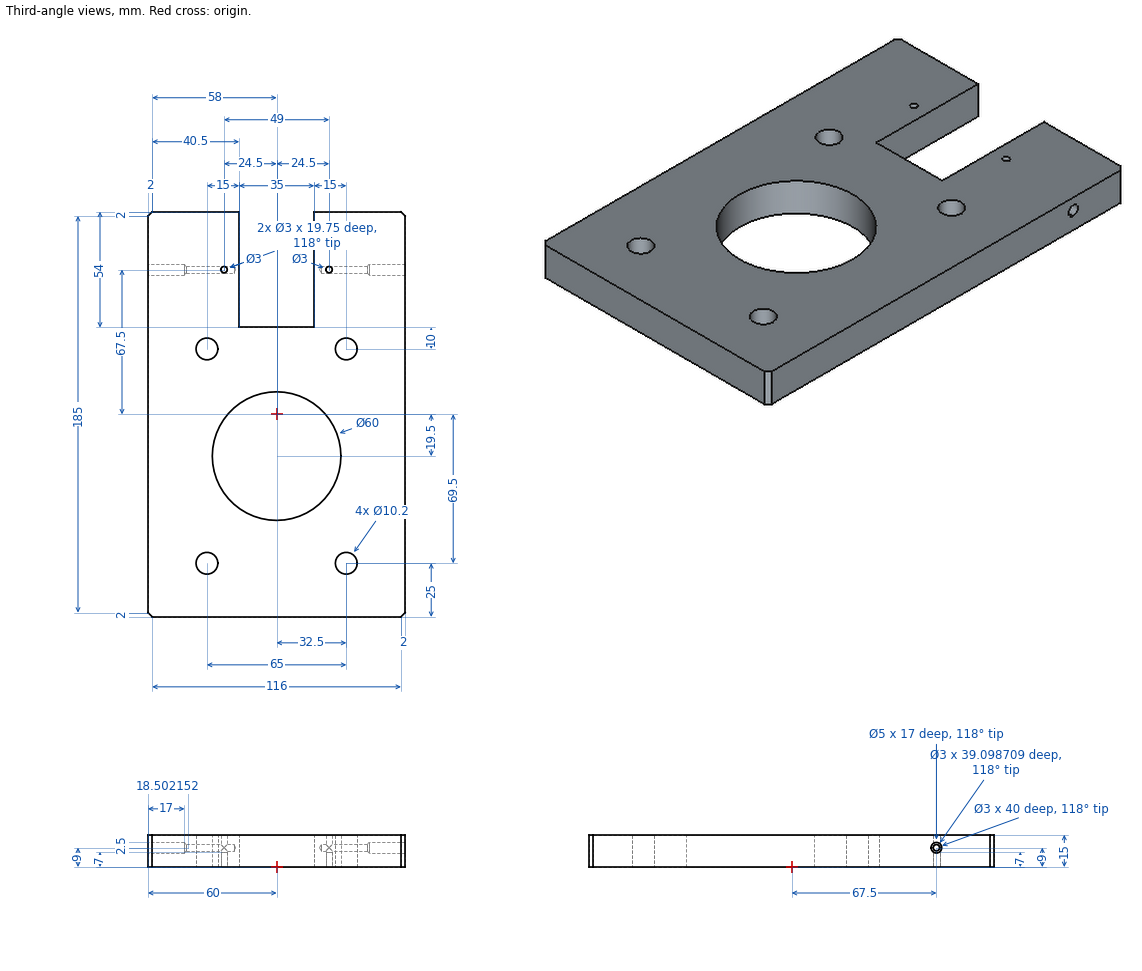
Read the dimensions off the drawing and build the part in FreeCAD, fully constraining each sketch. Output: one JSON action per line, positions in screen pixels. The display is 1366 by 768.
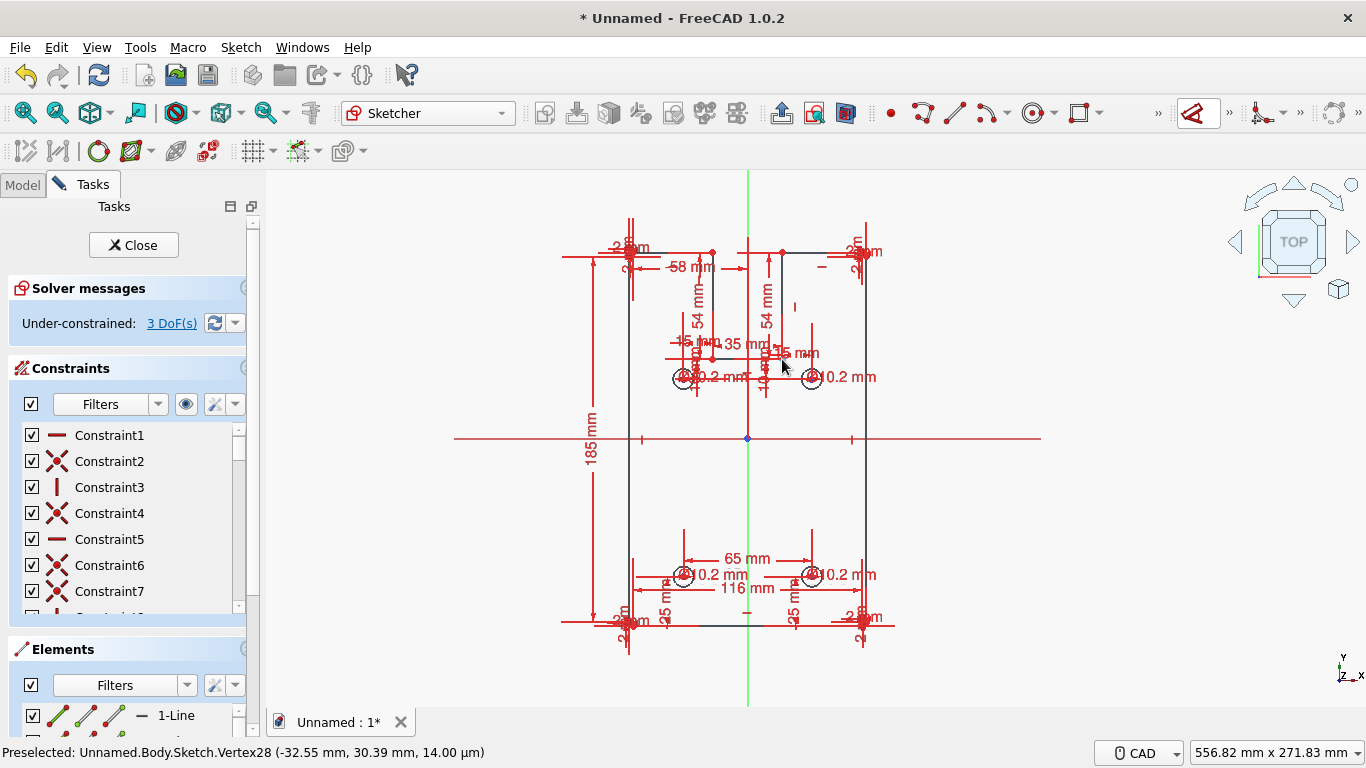
{"action": "left_click", "coordinate": [689, 253]}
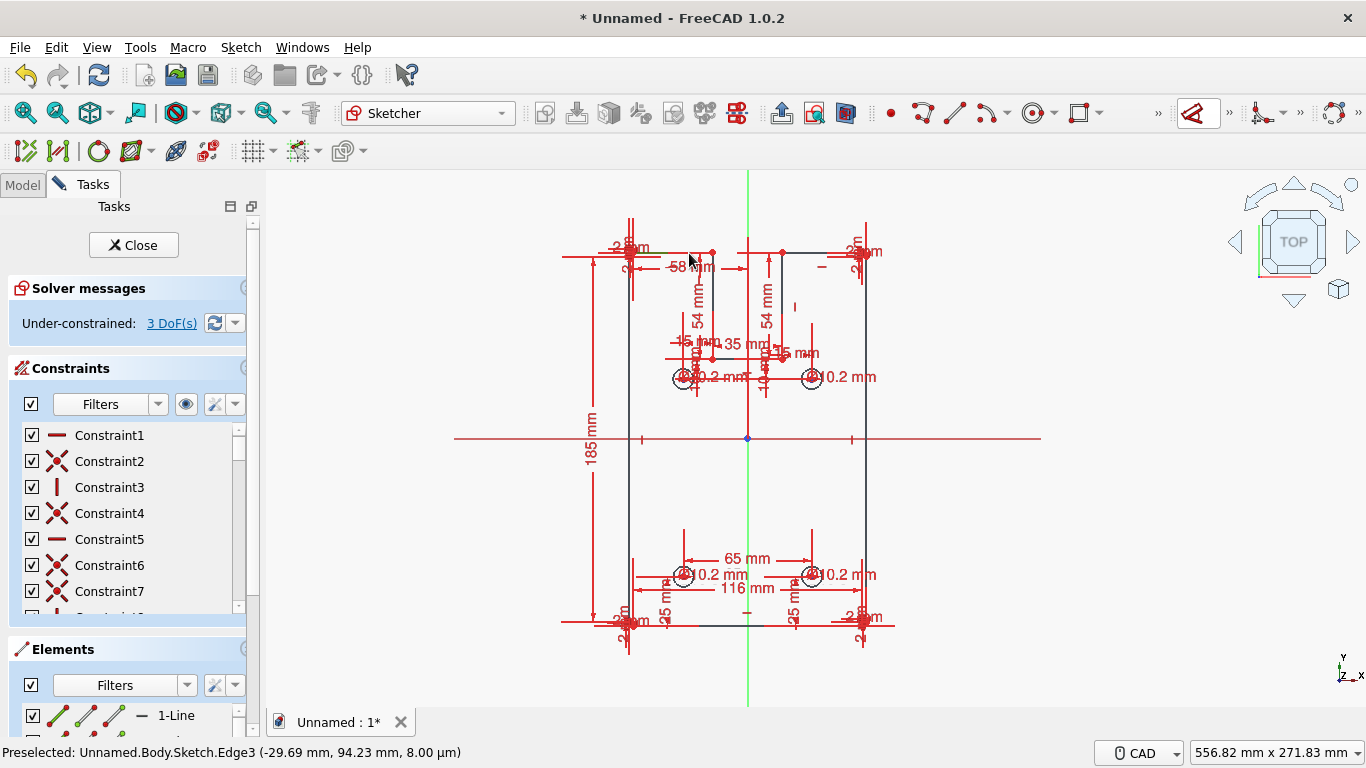
{"action": "key", "text": "l"}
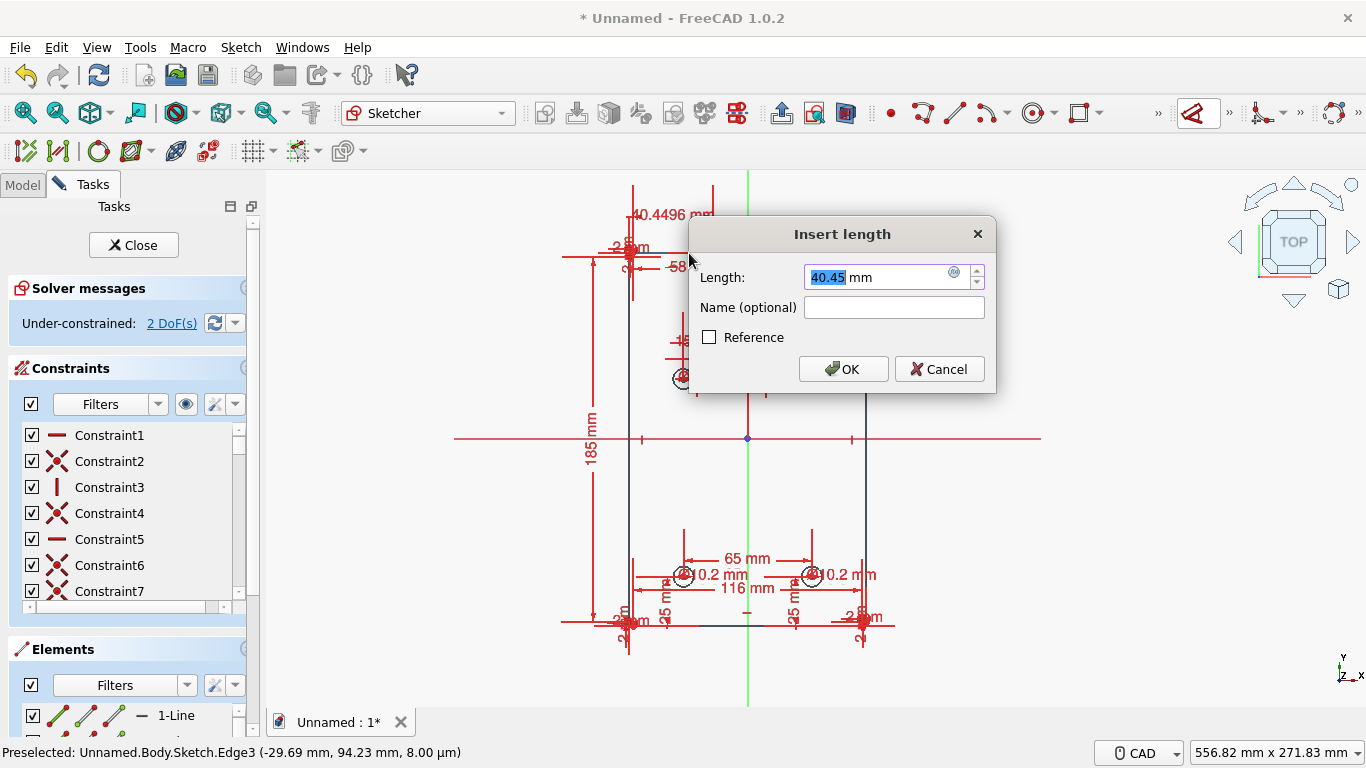
{"action": "type", "text": "40.5"}
{"action": "key", "text": "Return"}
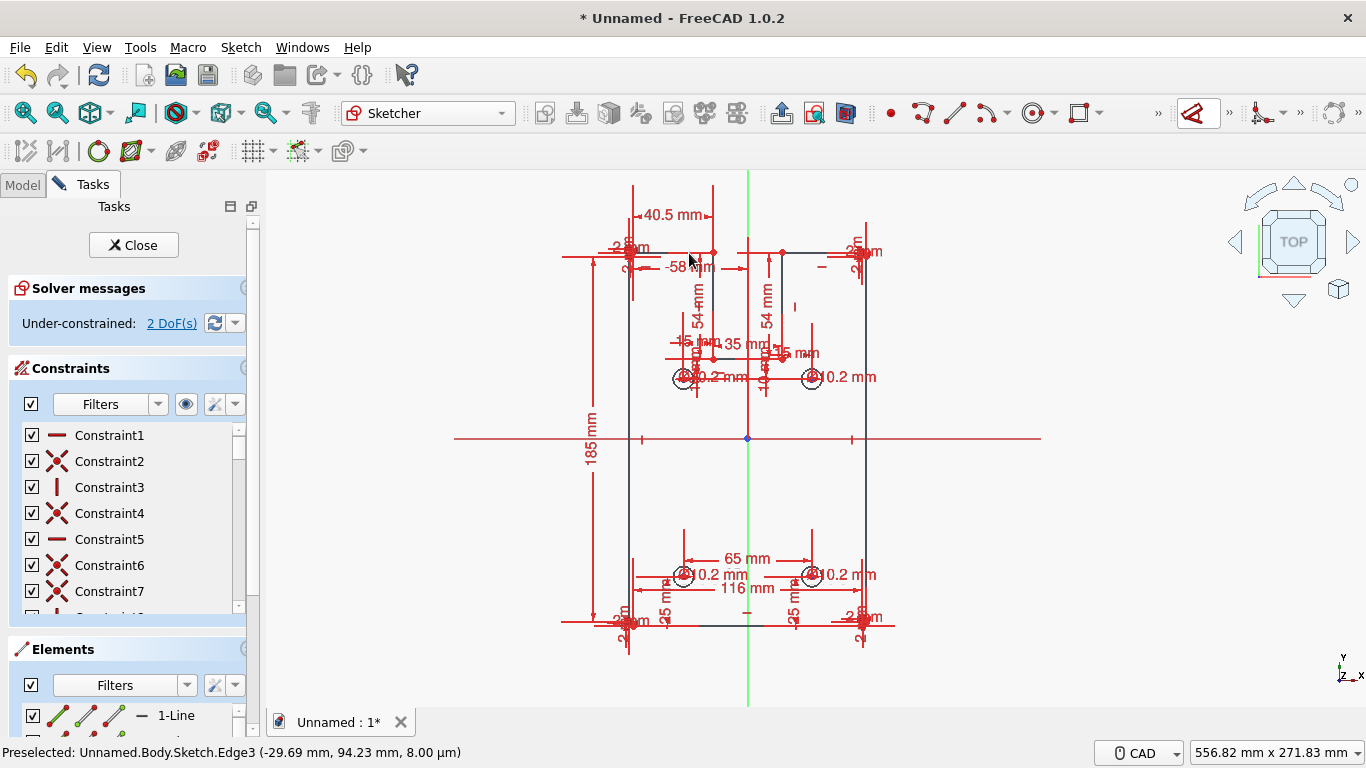
{"action": "left_click", "coordinate": [812, 577]}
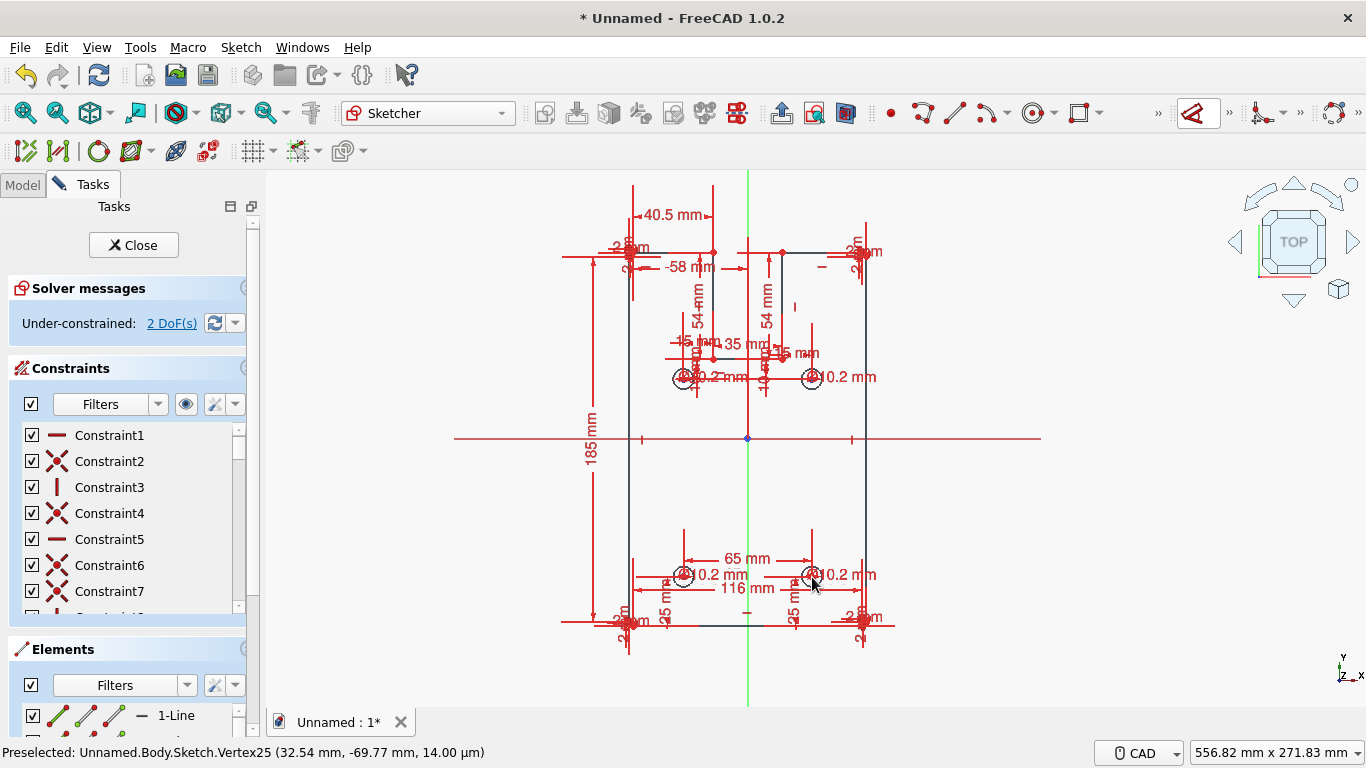
{"action": "key", "text": "l"}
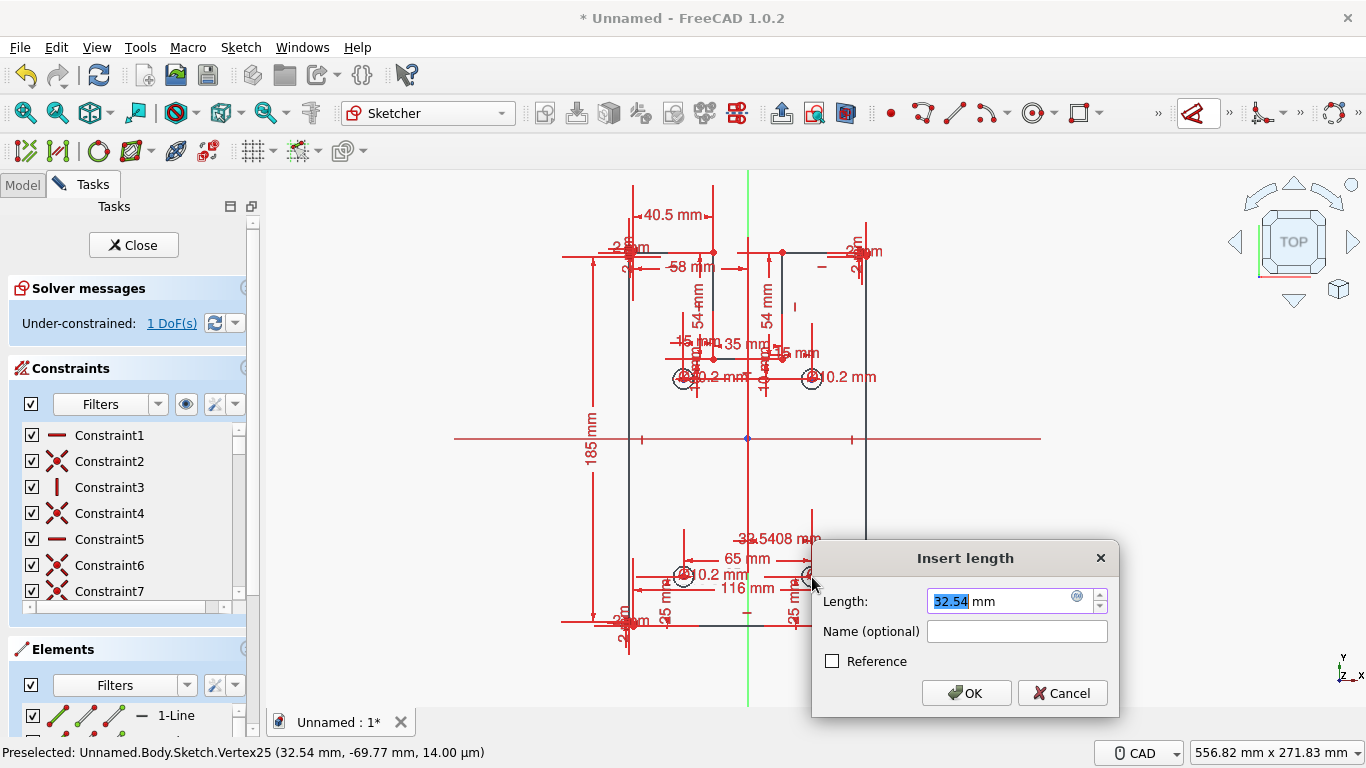
{"action": "type", "text": "32.5"}
{"action": "key", "text": "Return"}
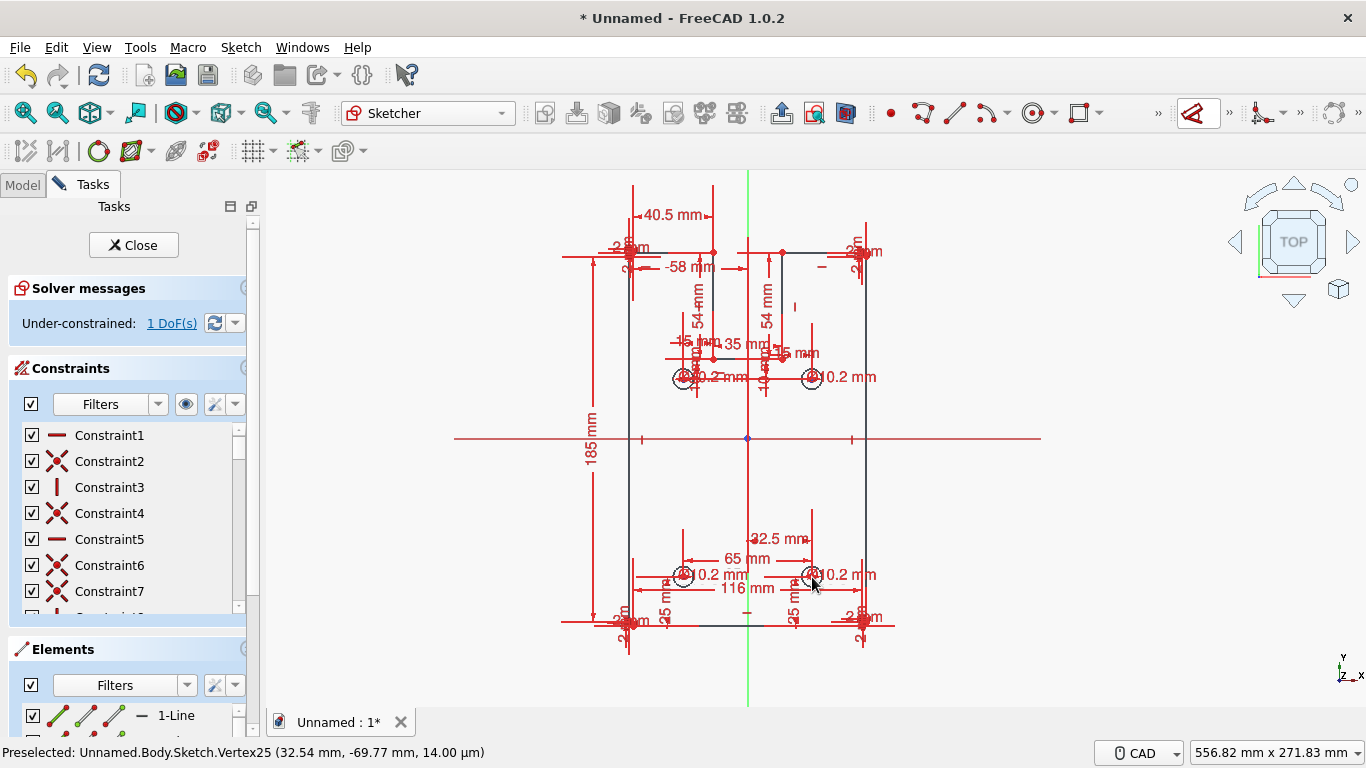
{"action": "left_click", "coordinate": [812, 577]}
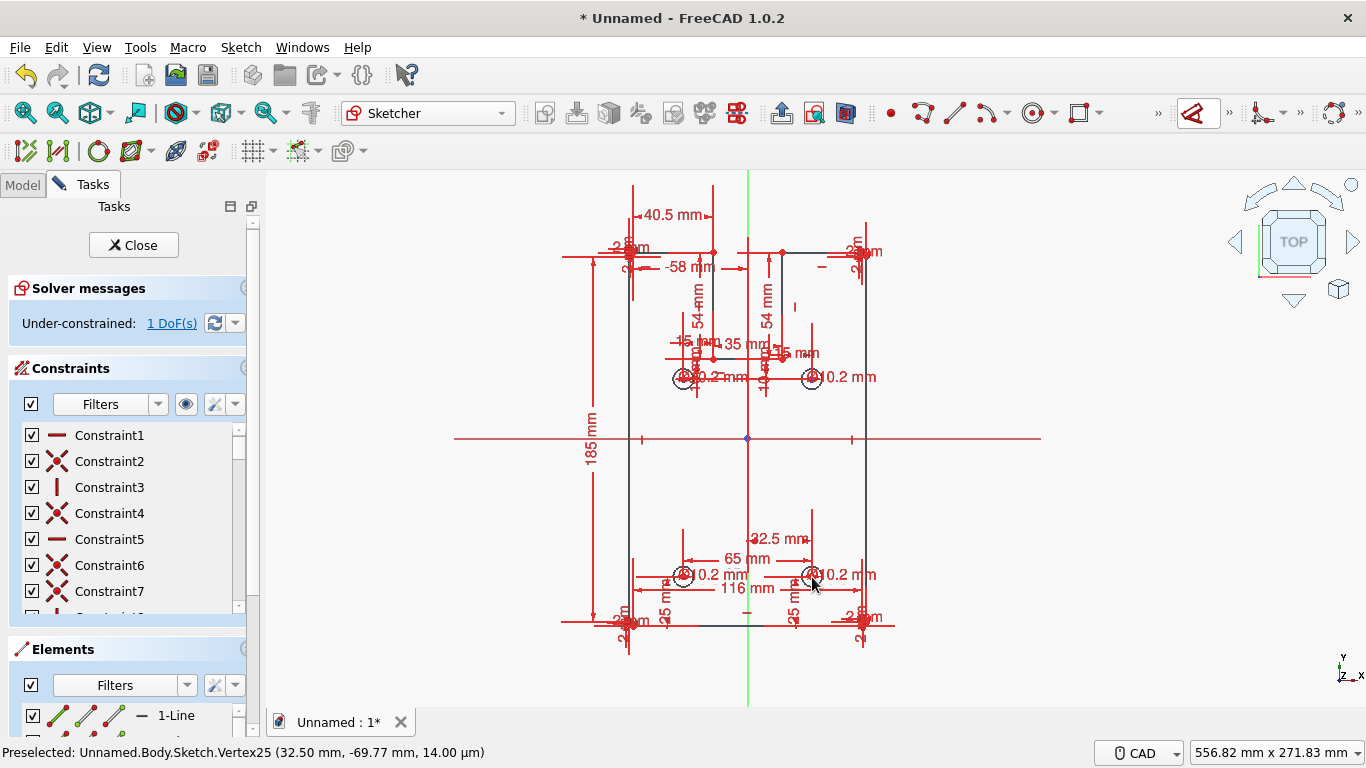
{"action": "key", "text": "i"}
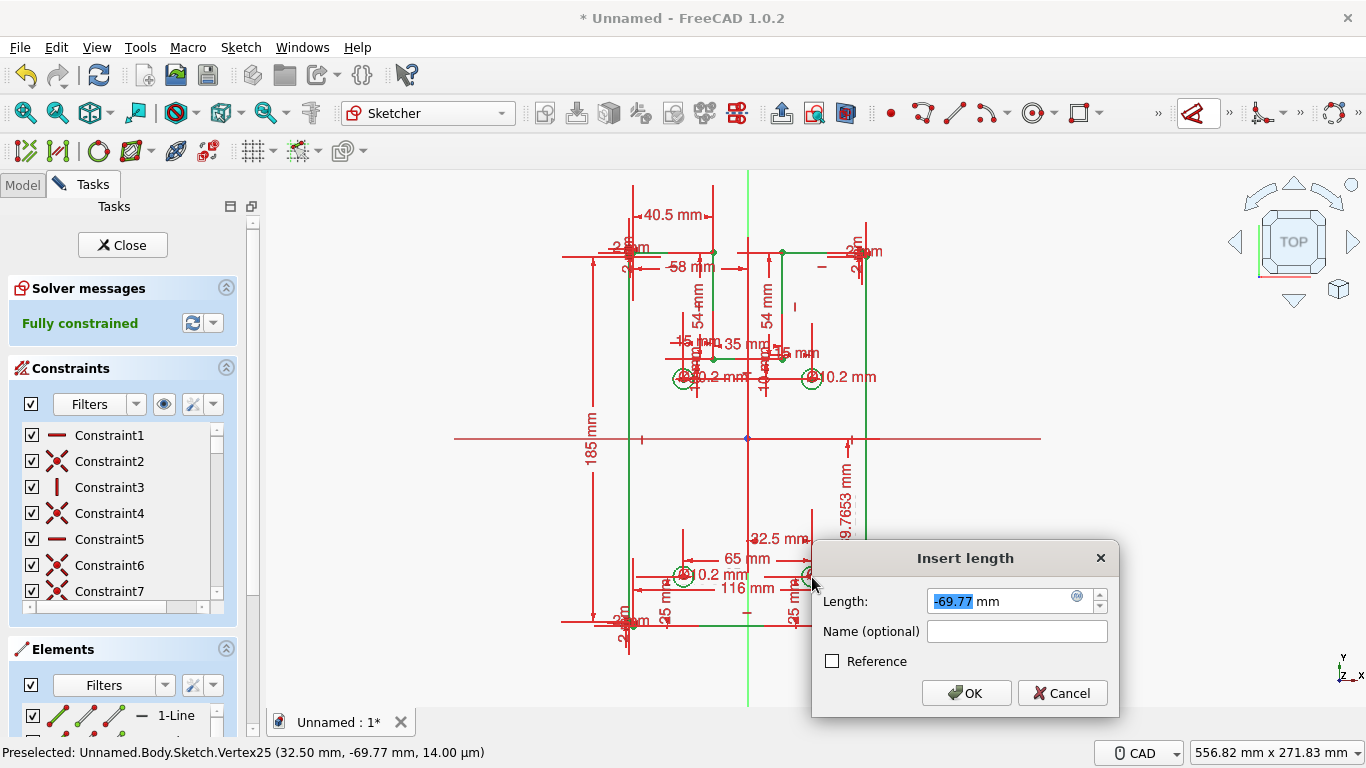
{"action": "type", "text": "-69.5"}
{"action": "key", "text": "Return"}